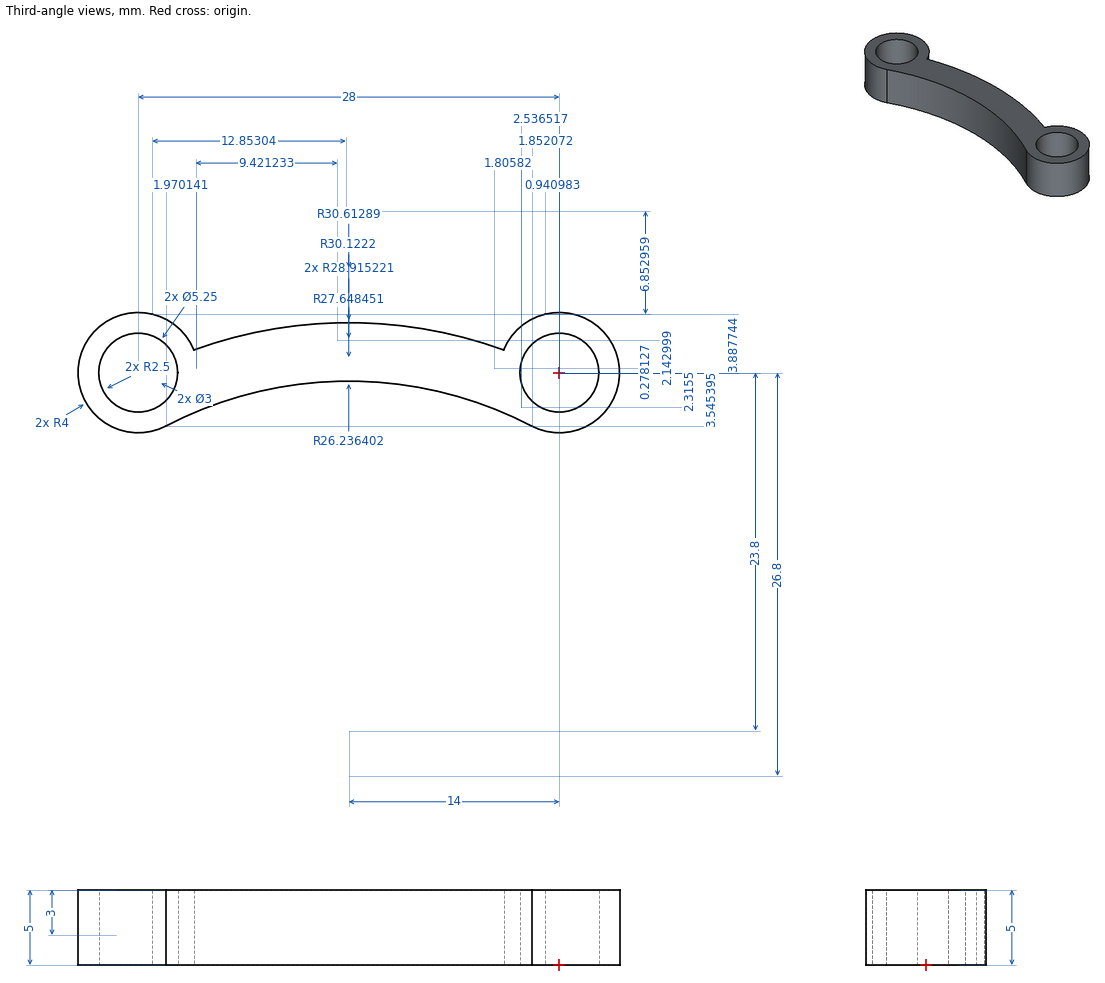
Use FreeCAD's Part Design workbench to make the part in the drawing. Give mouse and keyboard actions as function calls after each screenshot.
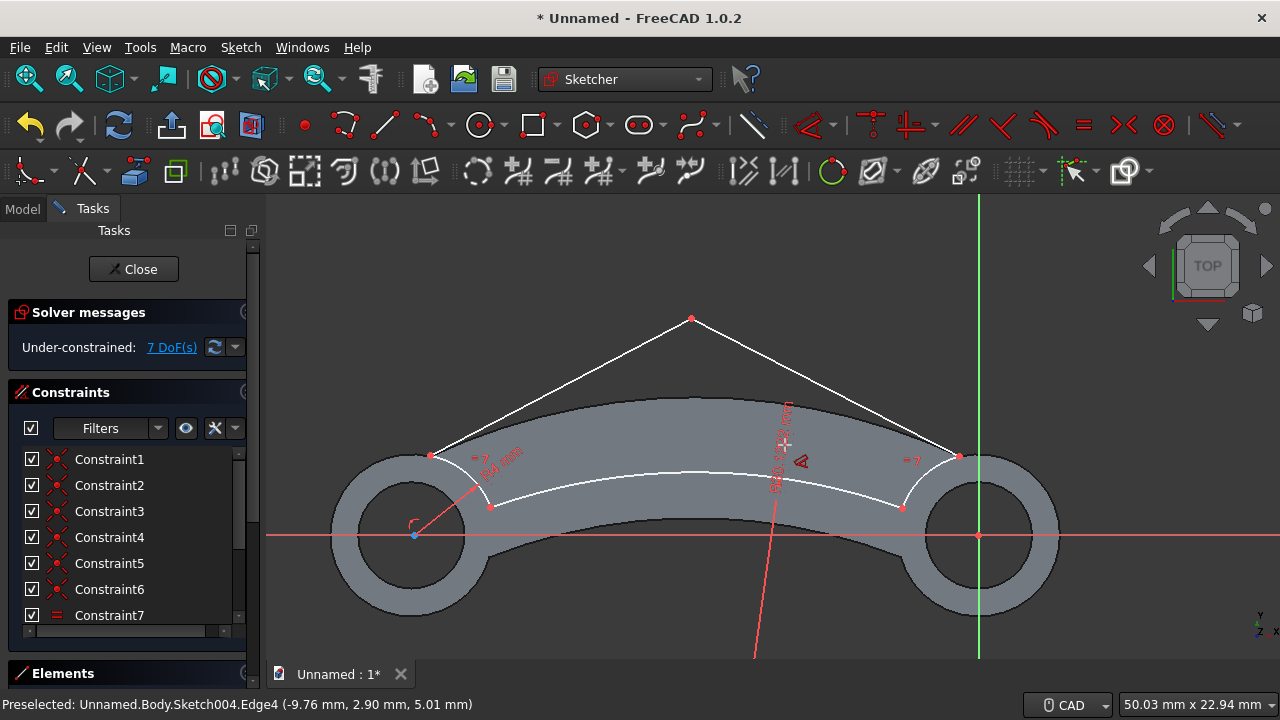
click(415, 535)
click(697, 569)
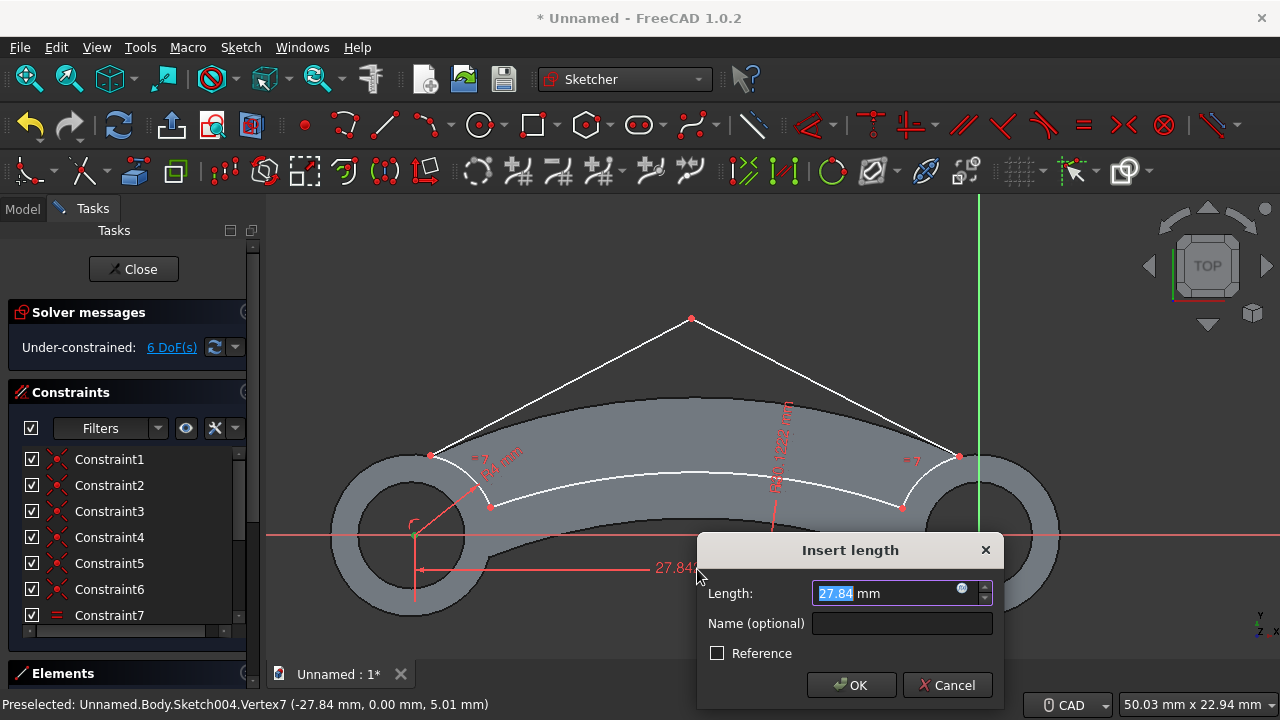
text(28)
key(Return)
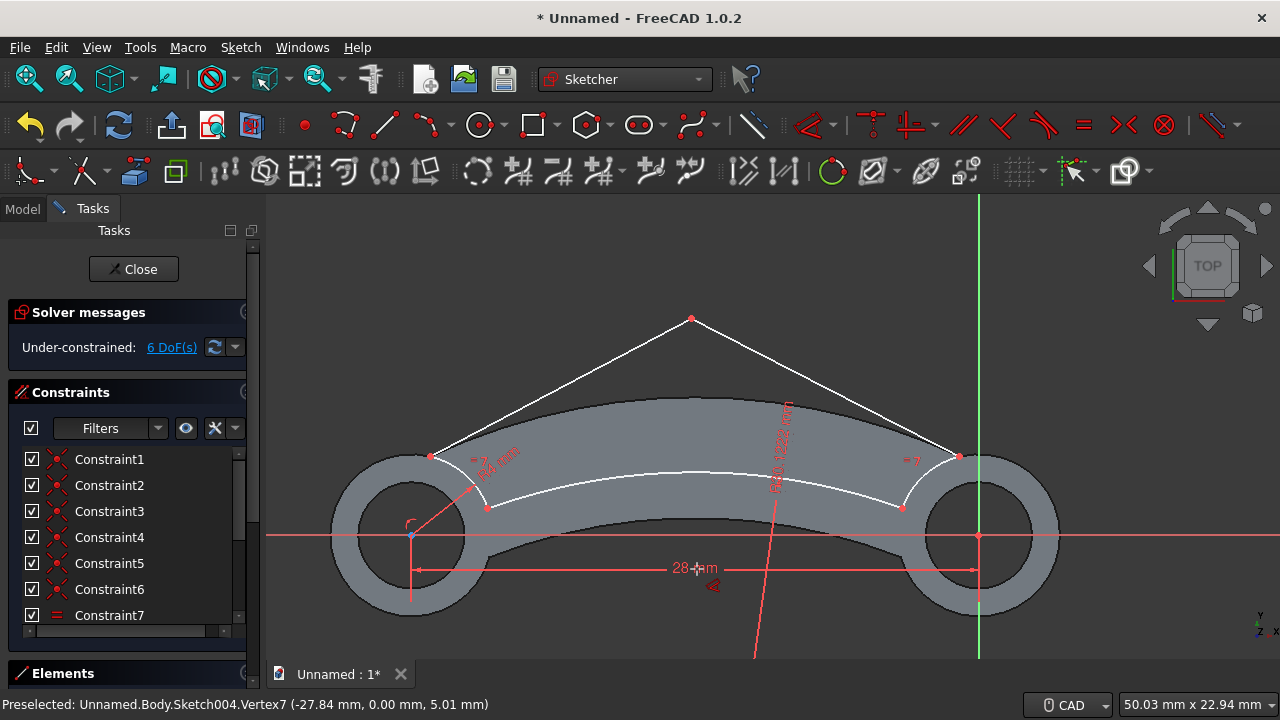
scroll(704, 267, down, 5)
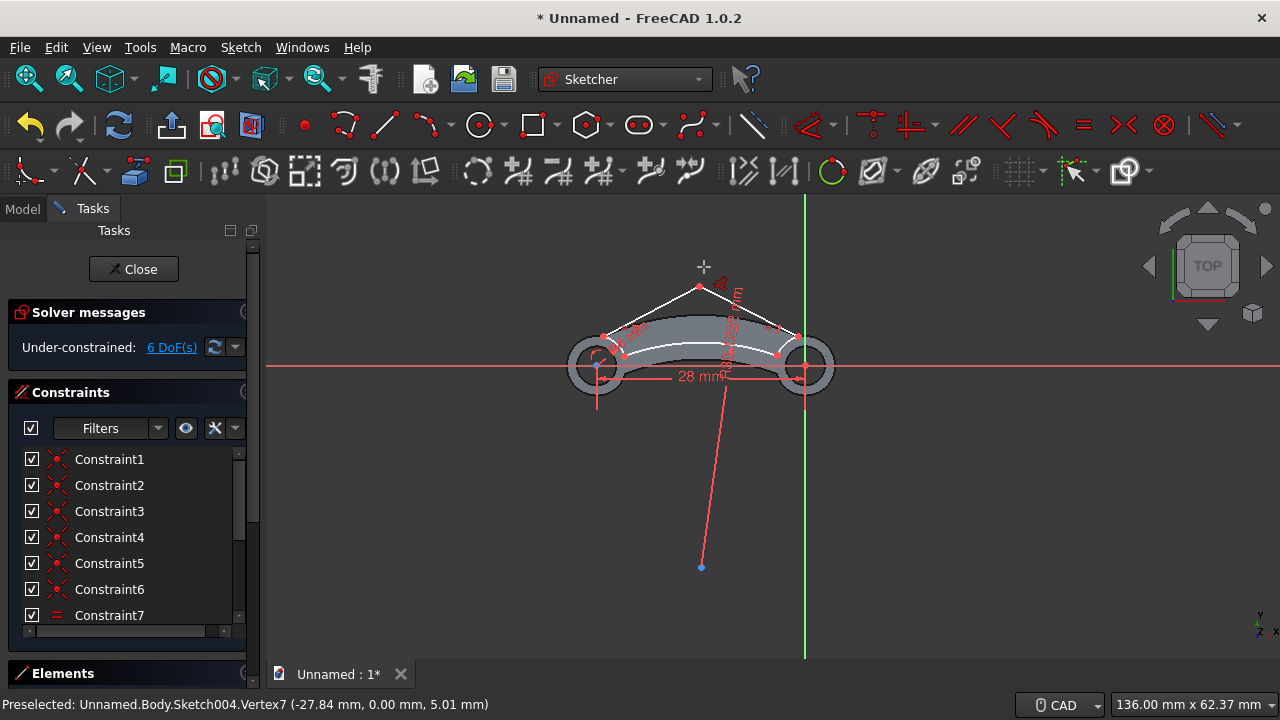
click(701, 567)
click(753, 601)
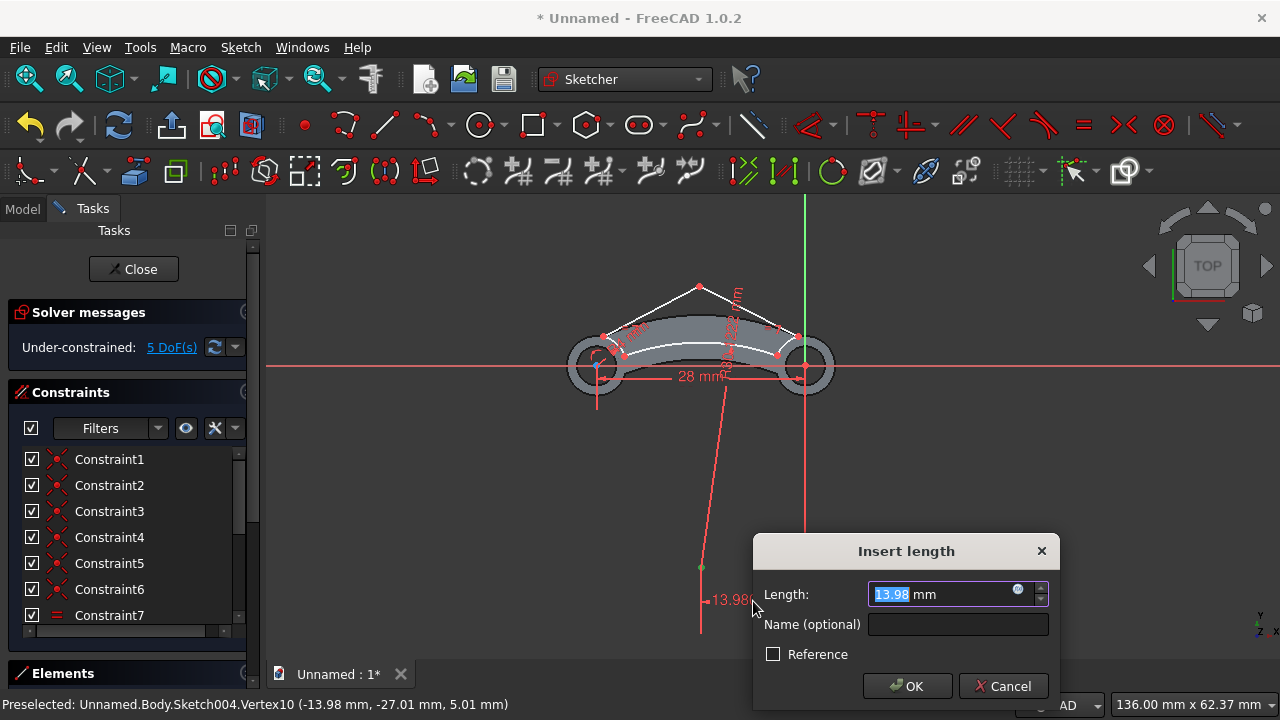
text(14)
key(Return)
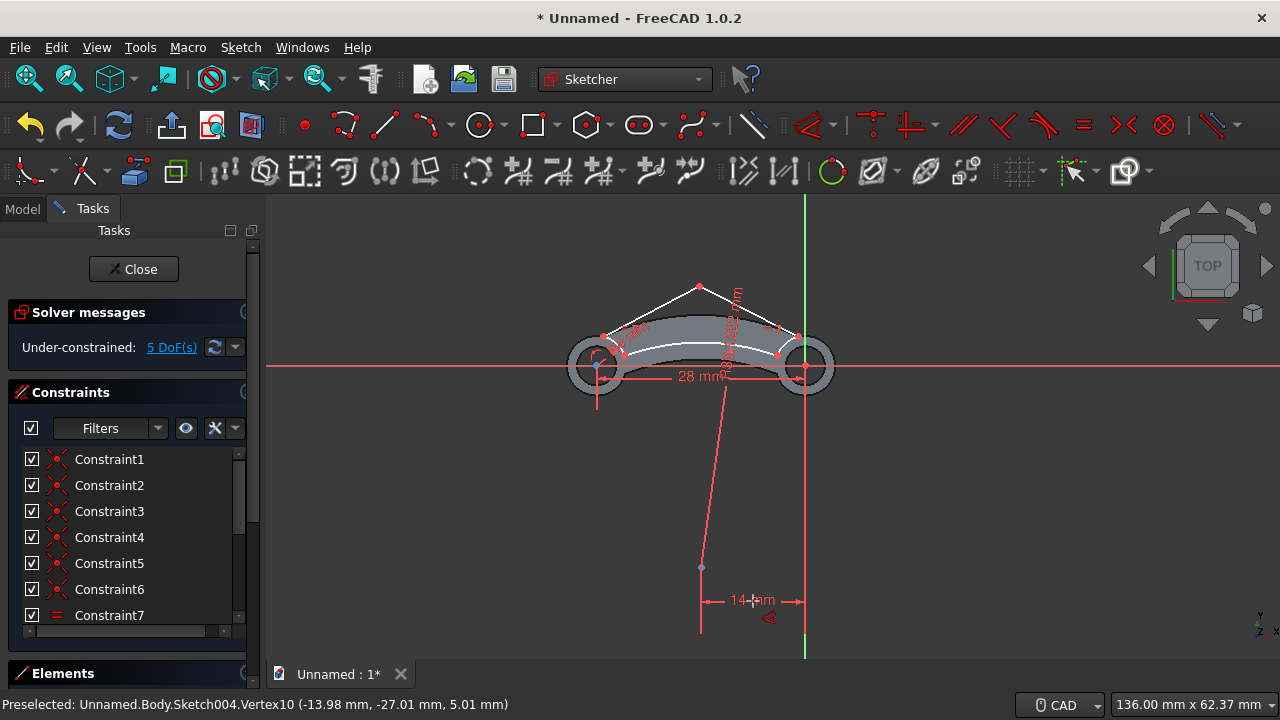
click(701, 567)
click(839, 467)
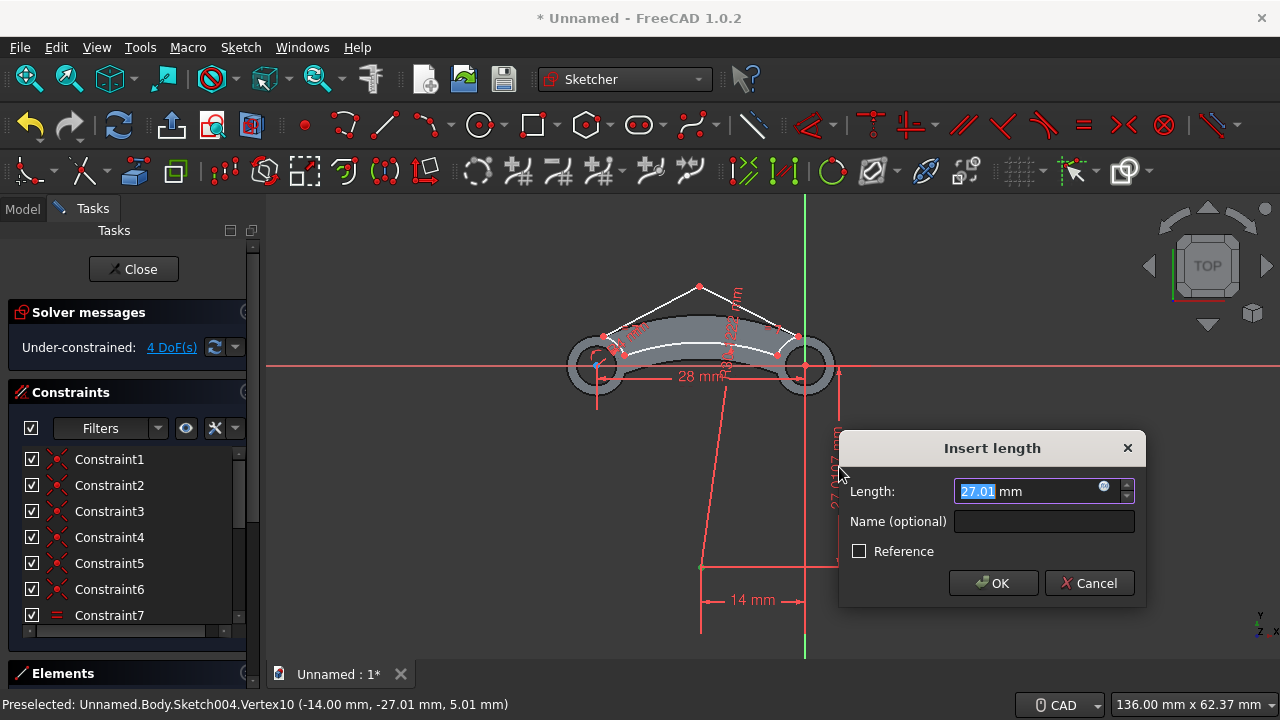
text(26.8)
key(Return)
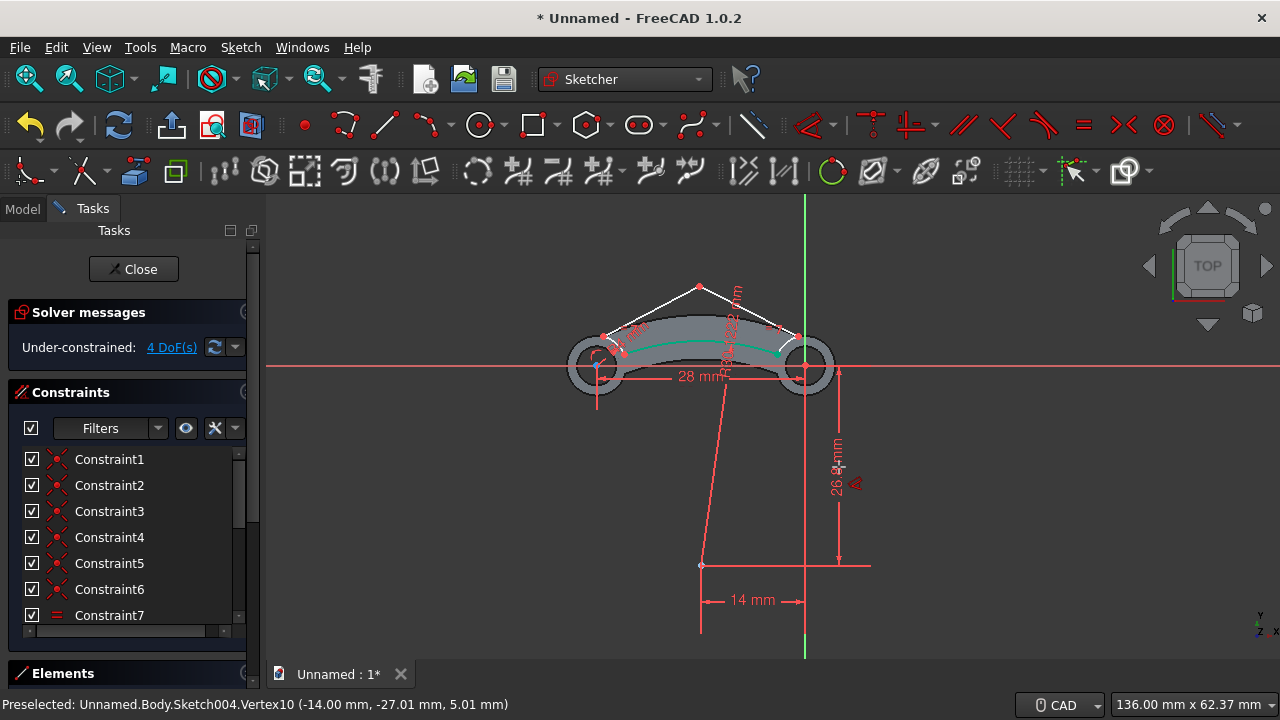
scroll(798, 337, up, 9)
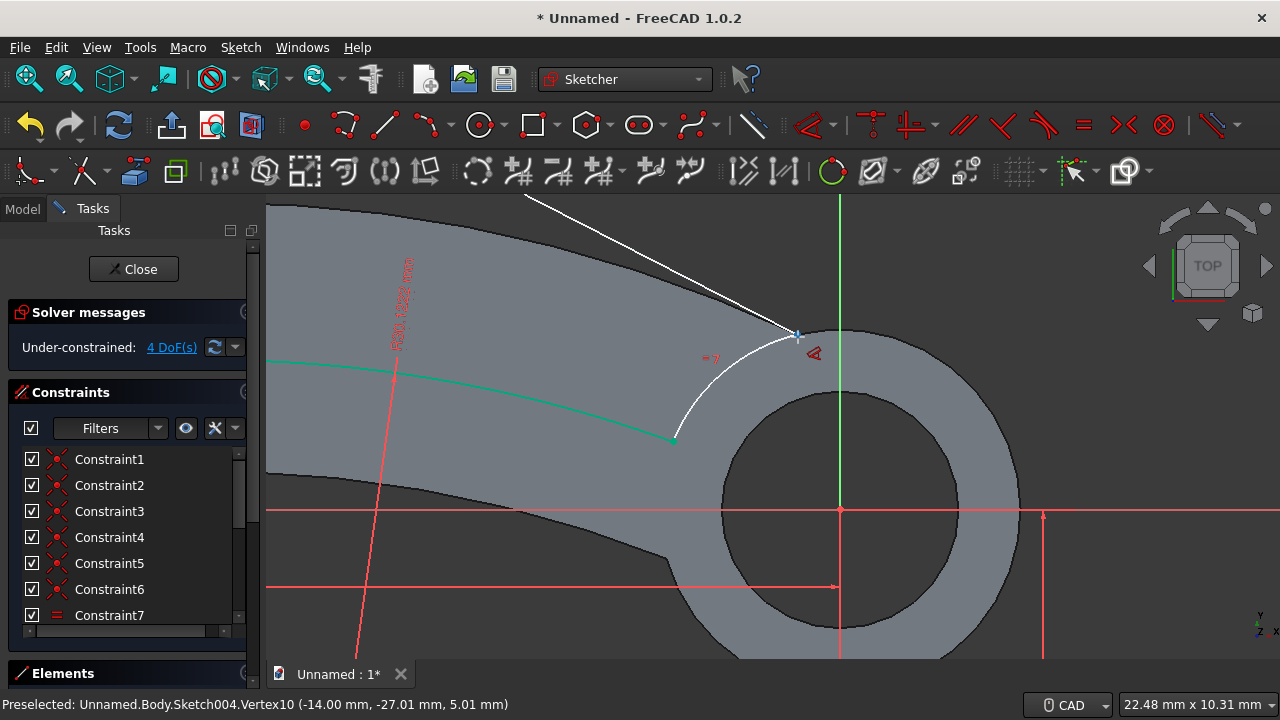
click(797, 335)
click(819, 544)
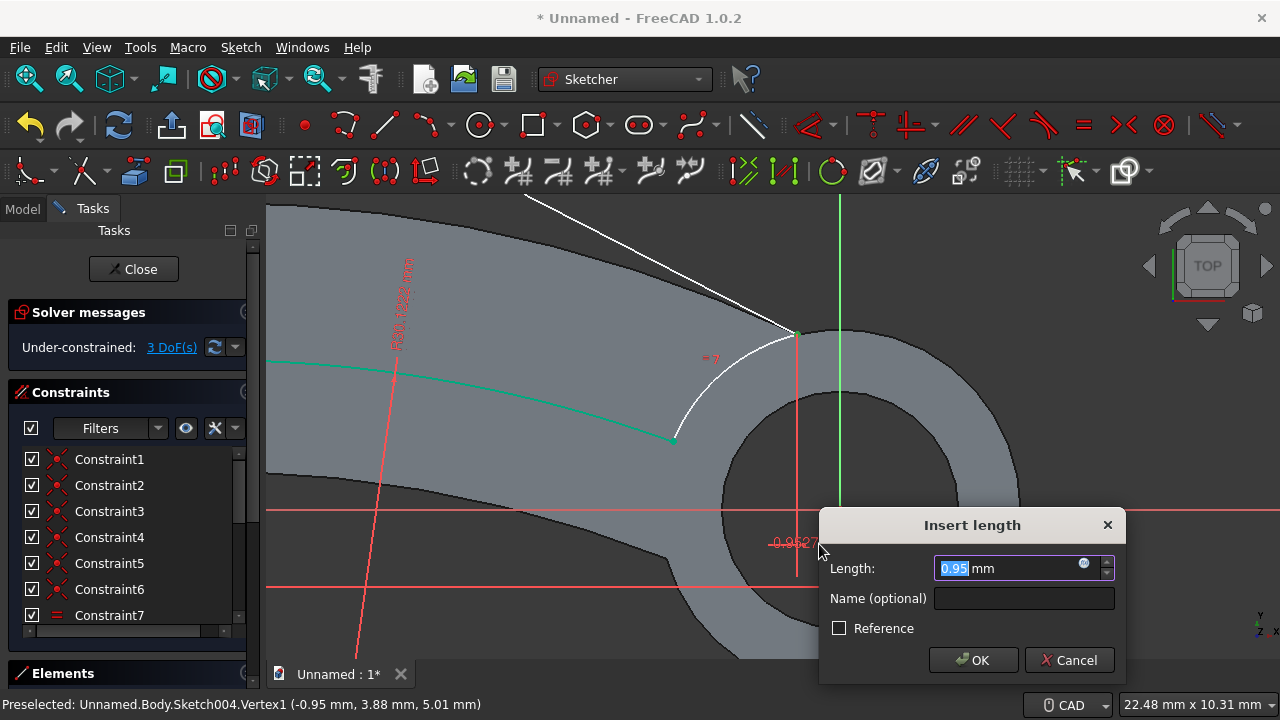
text(0.940983)
key(Return)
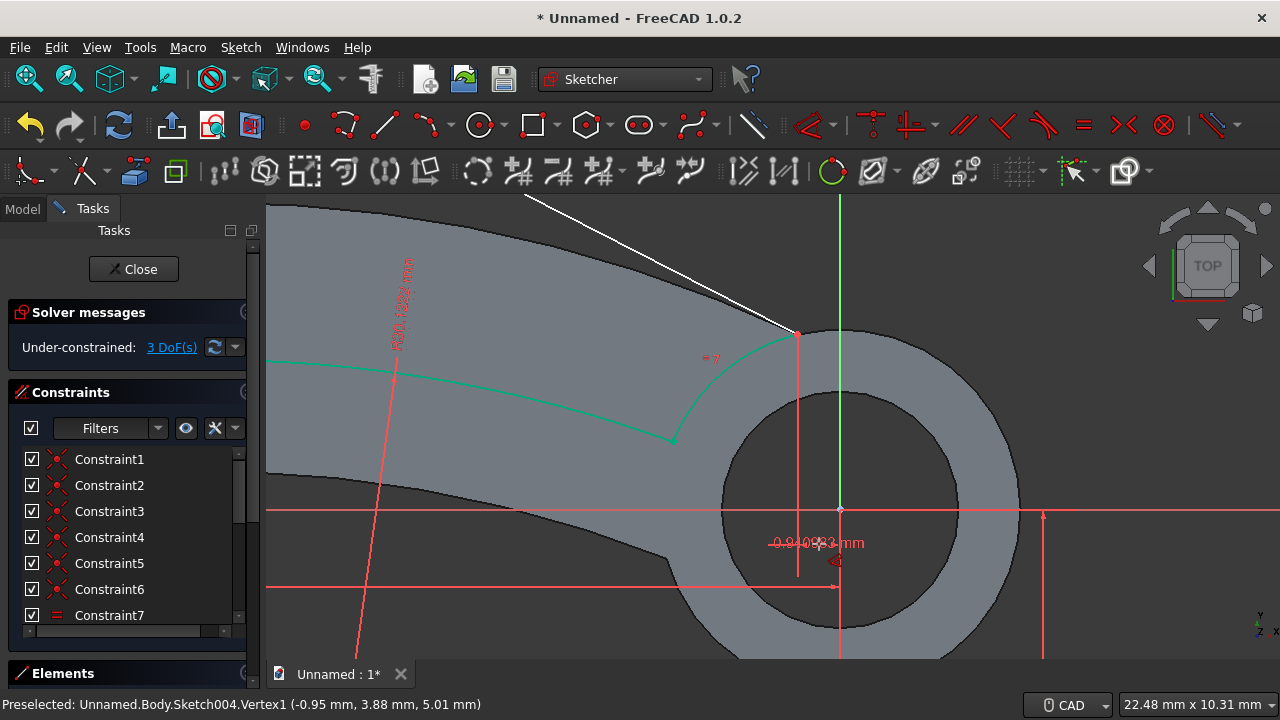
scroll(1092, 556, down, 4)